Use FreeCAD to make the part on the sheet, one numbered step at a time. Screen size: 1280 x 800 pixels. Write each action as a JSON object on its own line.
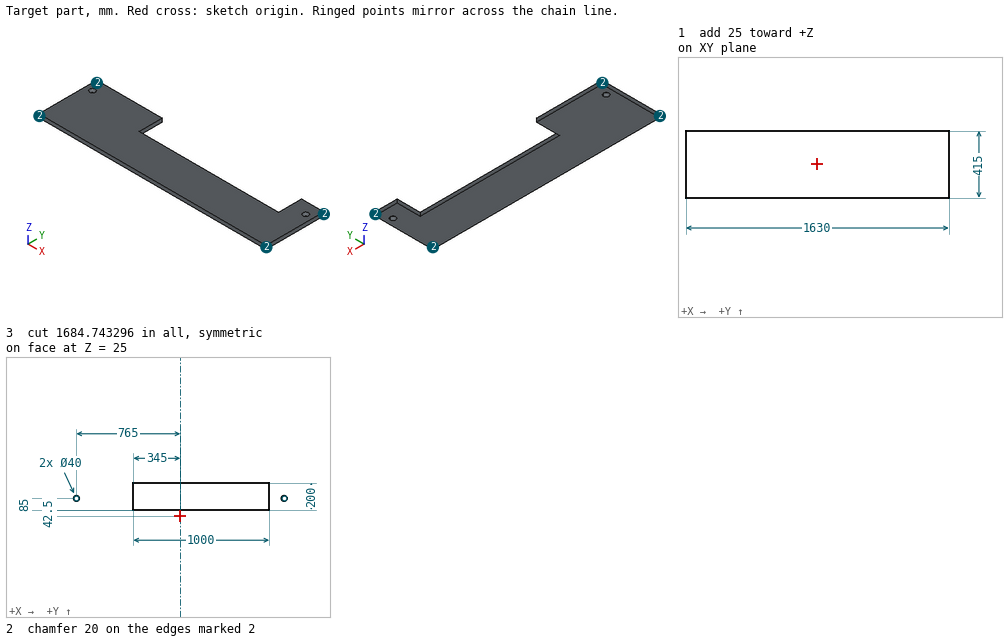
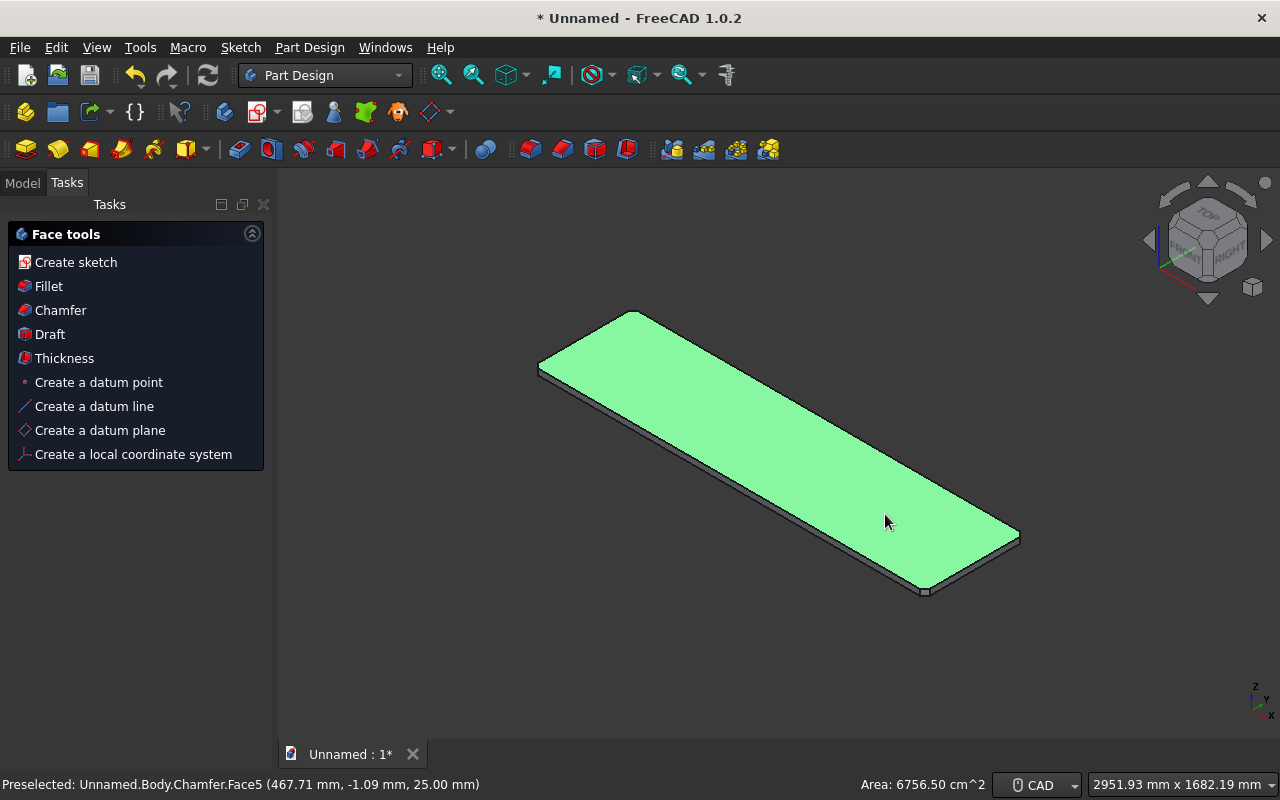
{"action": "left_click", "coordinate": [258, 112]}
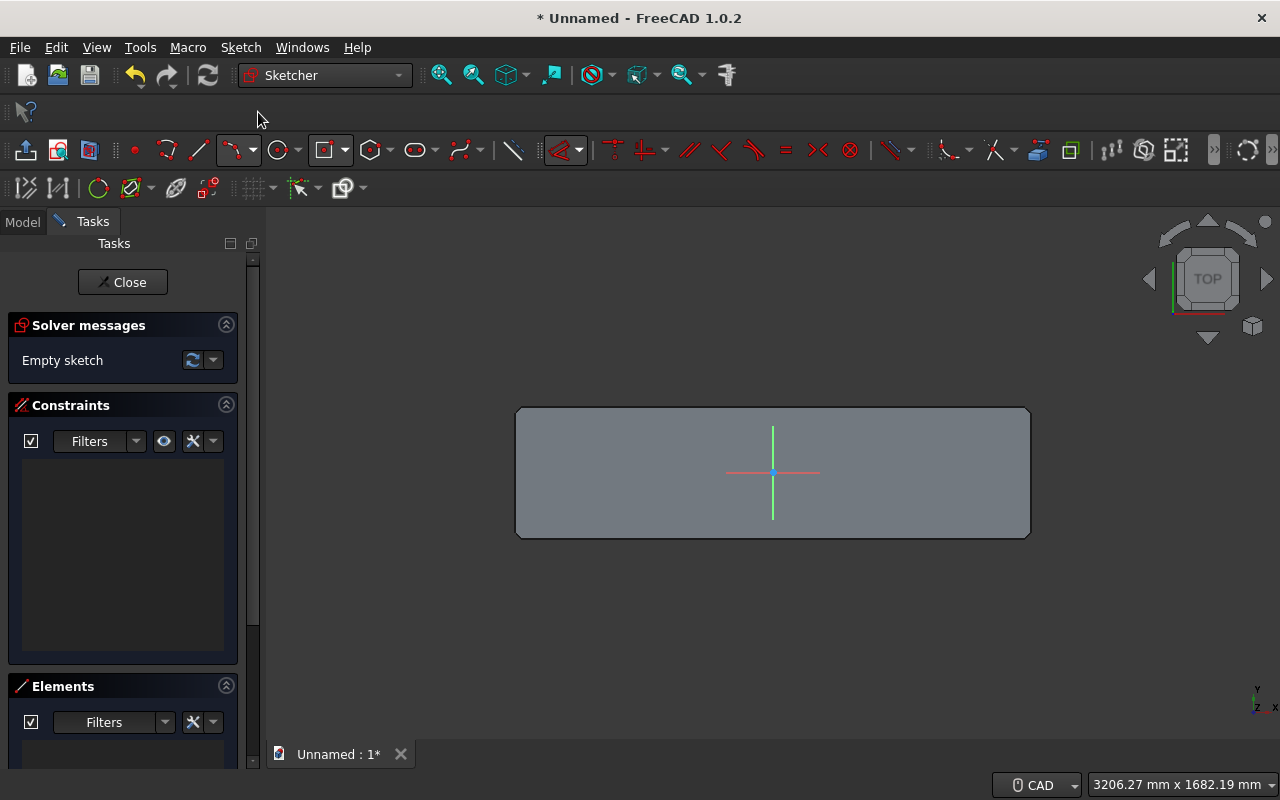
{"action": "key", "text": "g r"}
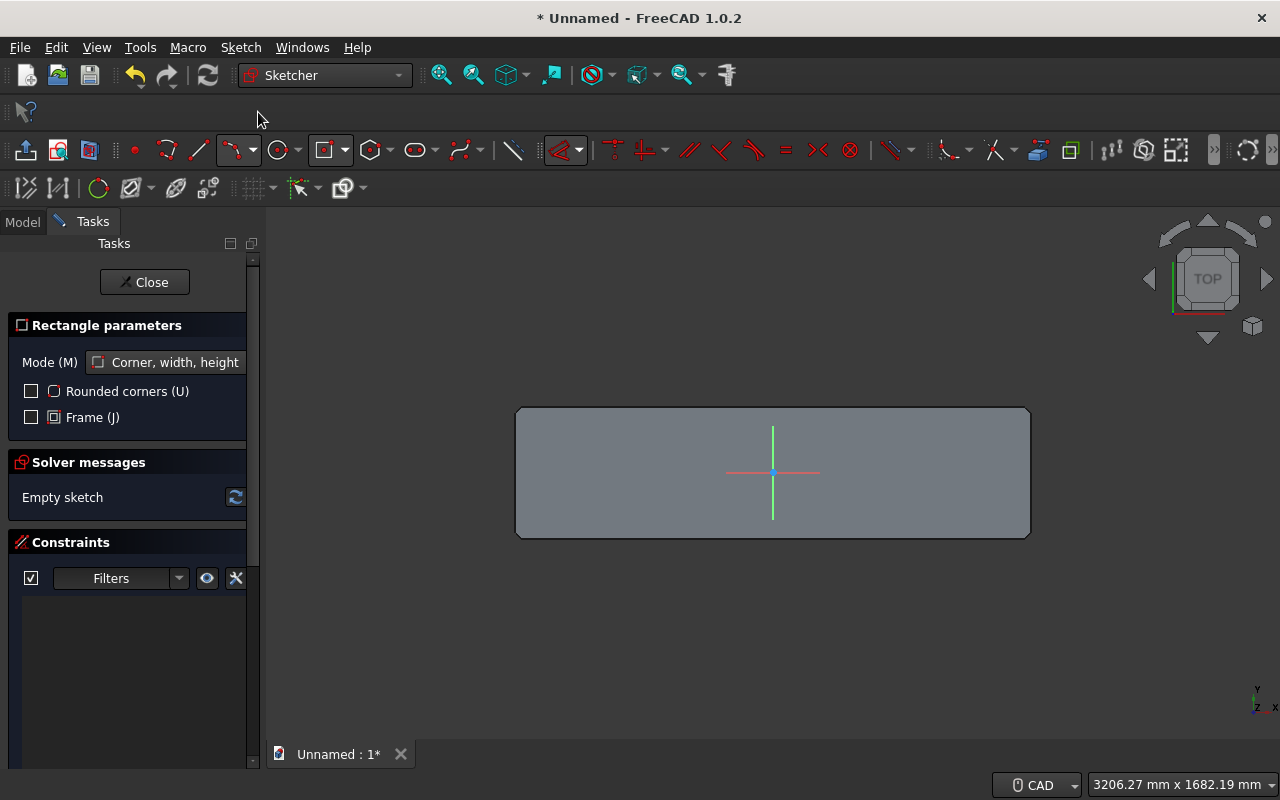
{"action": "left_click", "coordinate": [664, 396]}
{"action": "mouse_move", "coordinate": [980, 460]}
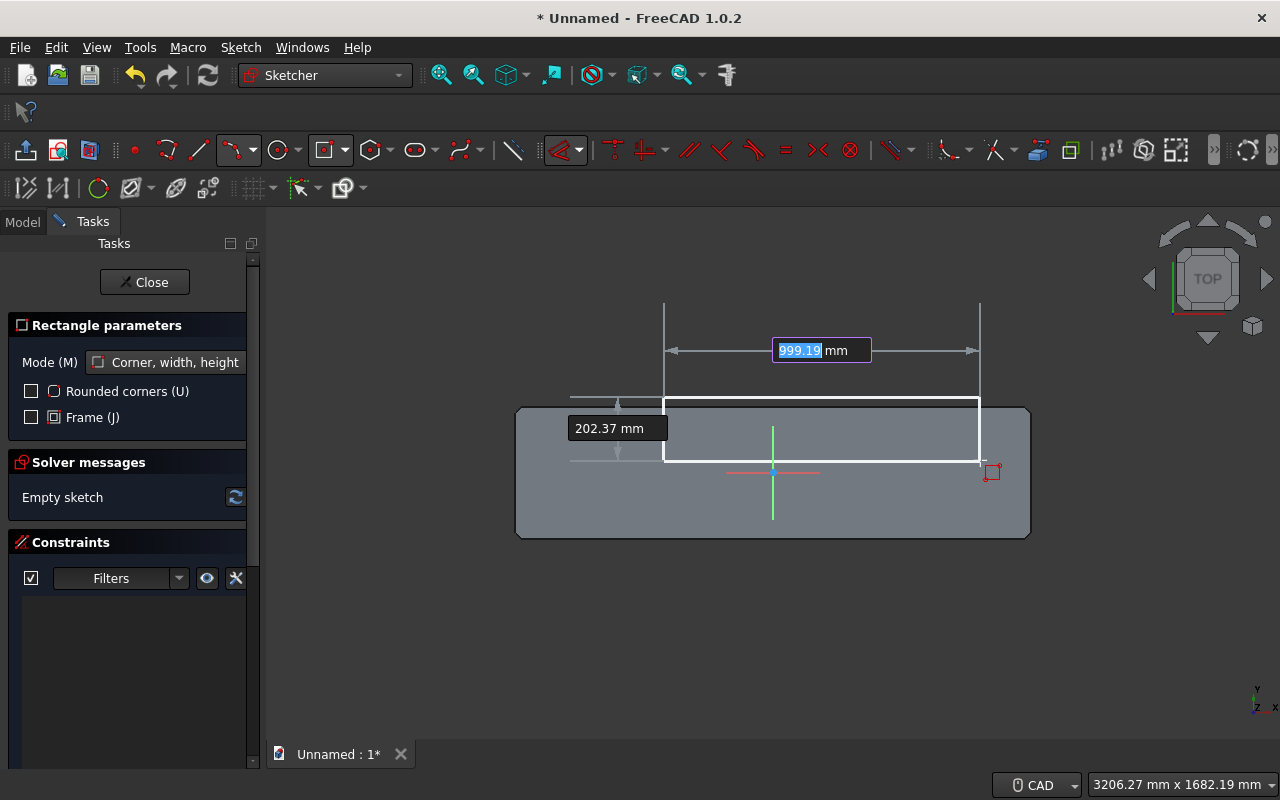
{"action": "type", "text": "1000"}
{"action": "key", "text": "Tab"}
{"action": "type", "text": "200"}
{"action": "key", "text": "Return"}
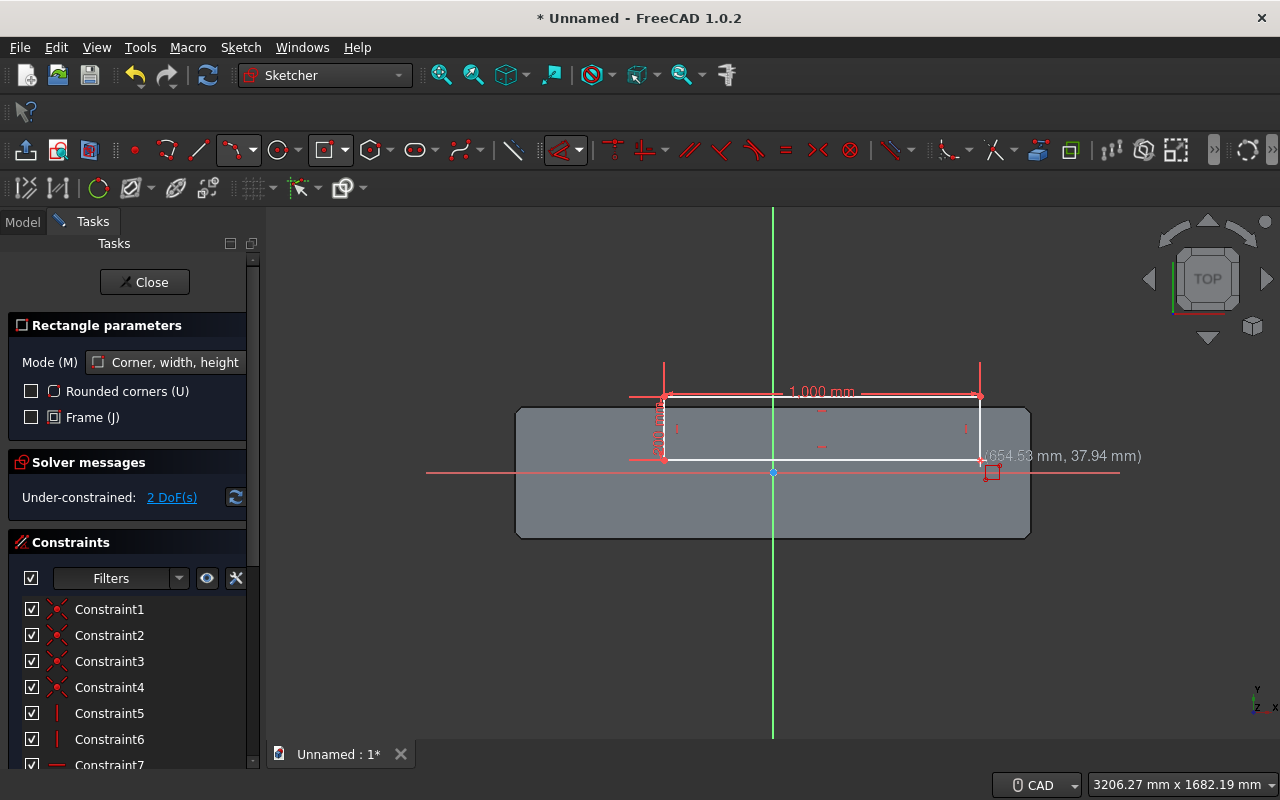
{"action": "left_click", "coordinate": [278, 150]}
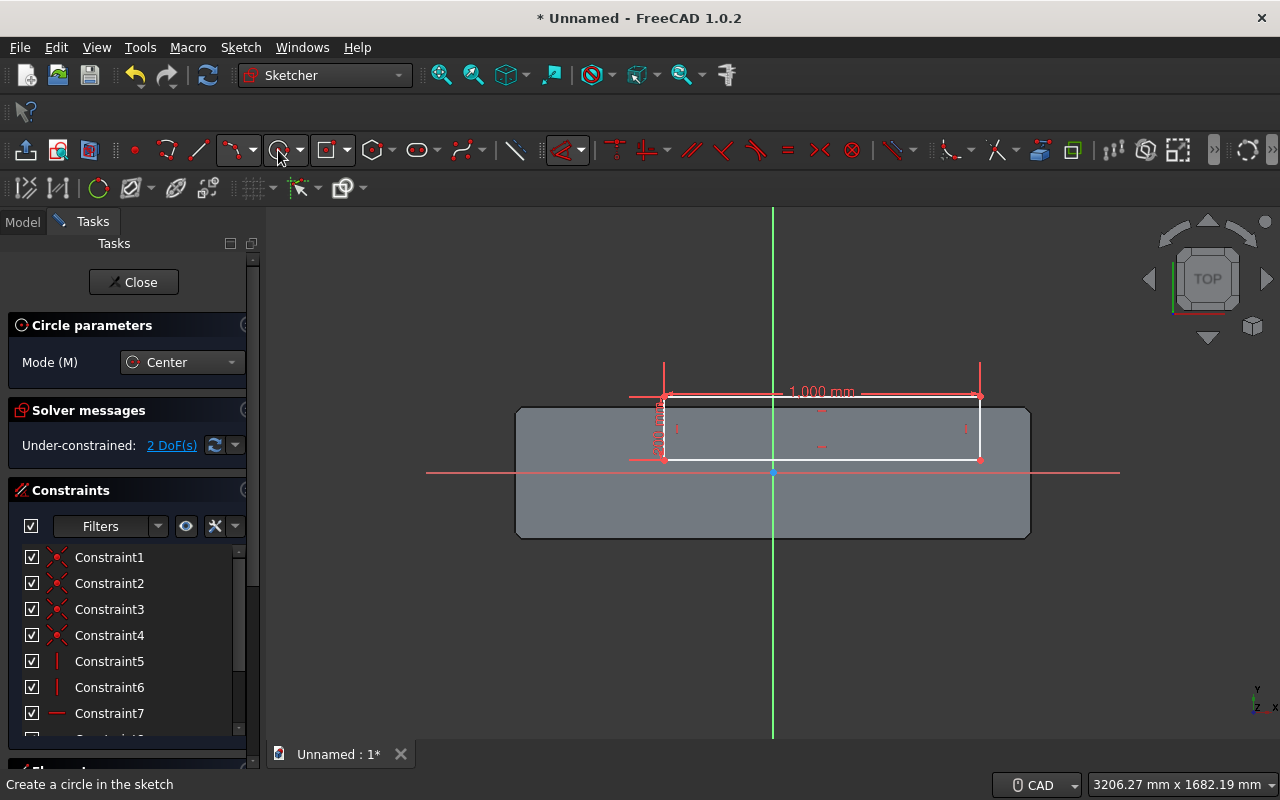
{"action": "scroll", "coordinate": [531, 433], "scroll_direction": "up", "scroll_amount": 7}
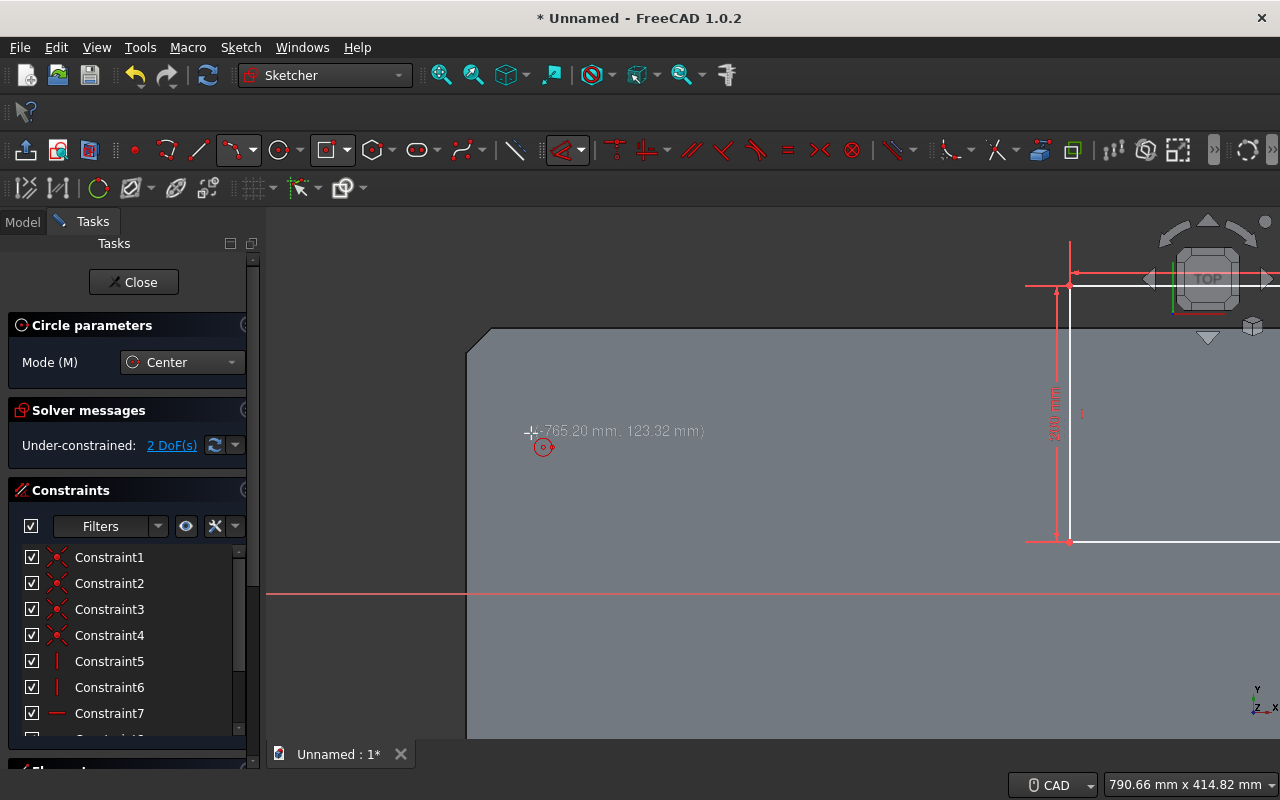
{"action": "scroll", "coordinate": [357, 488], "scroll_direction": "down", "scroll_amount": 6}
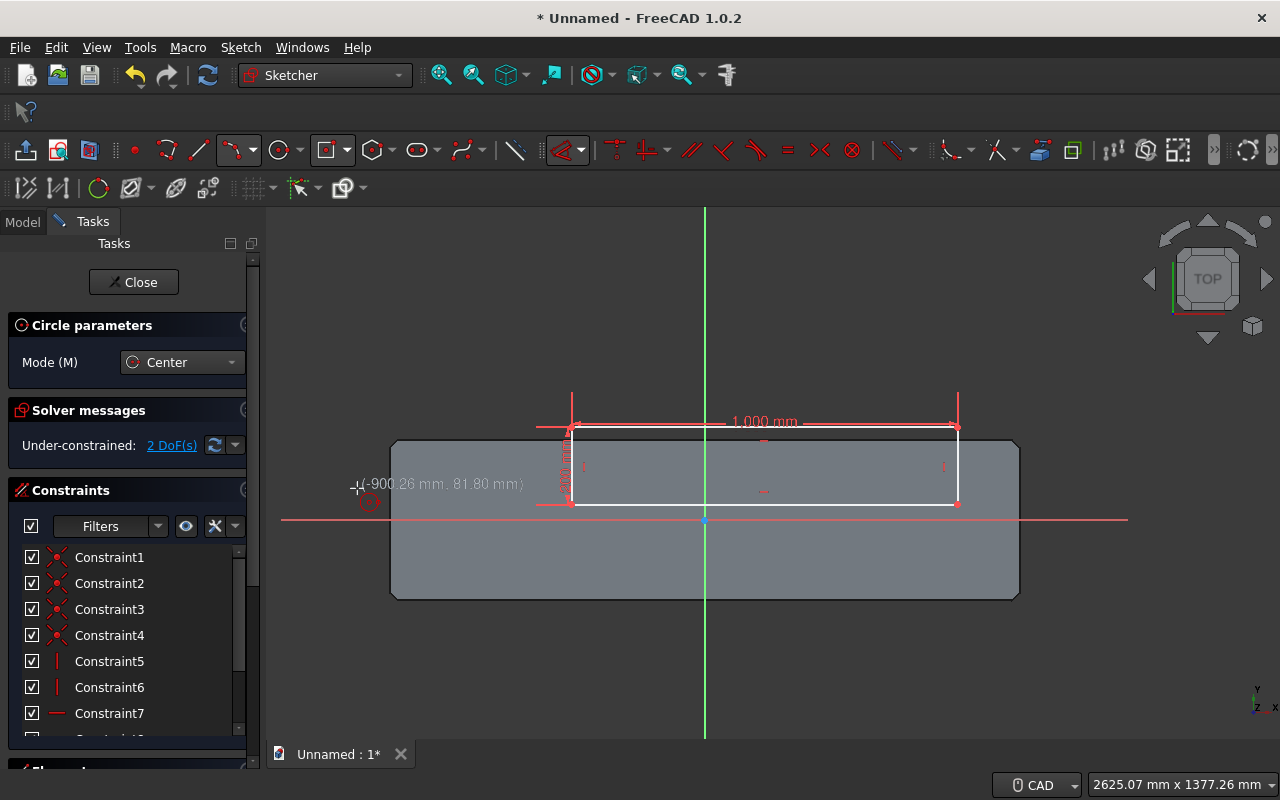
{"action": "left_click", "coordinate": [409, 471]}
{"action": "mouse_move", "coordinate": [415, 466]}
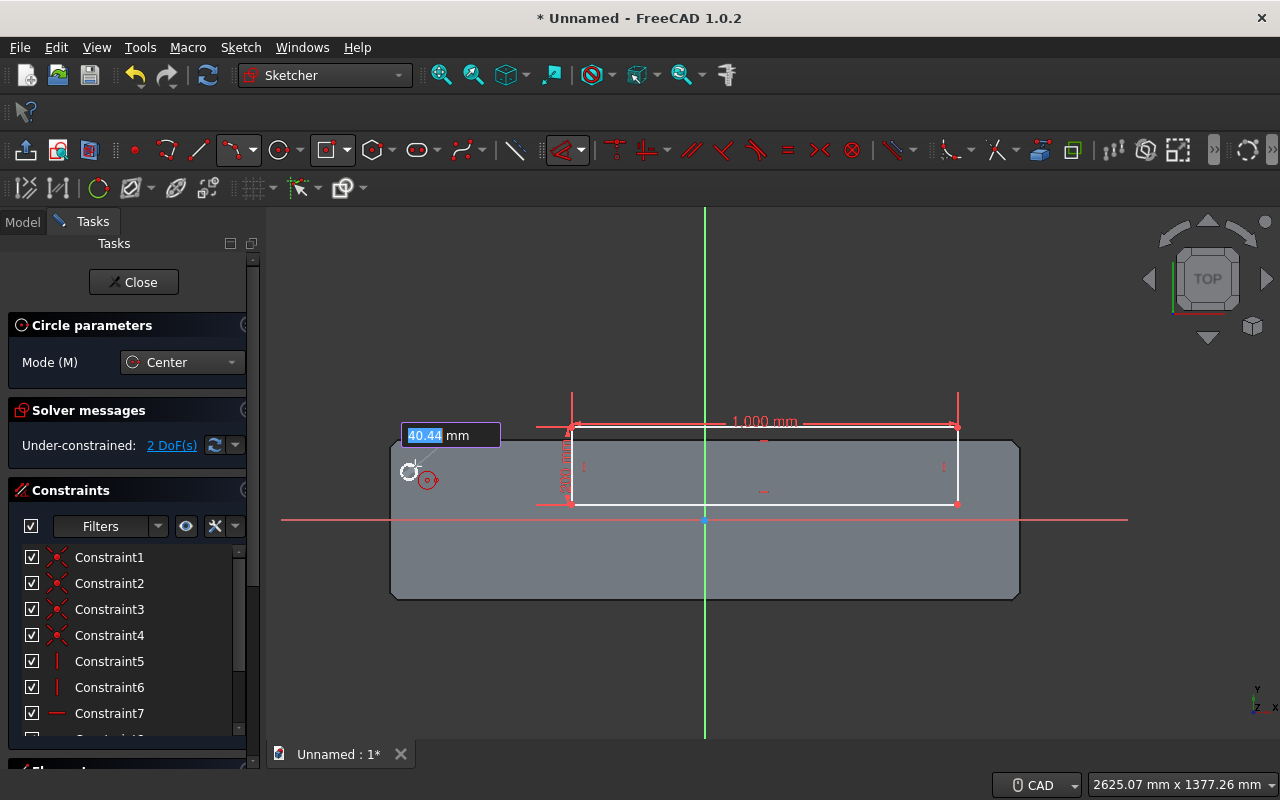
{"action": "type", "text": "40"}
{"action": "key", "text": "Return"}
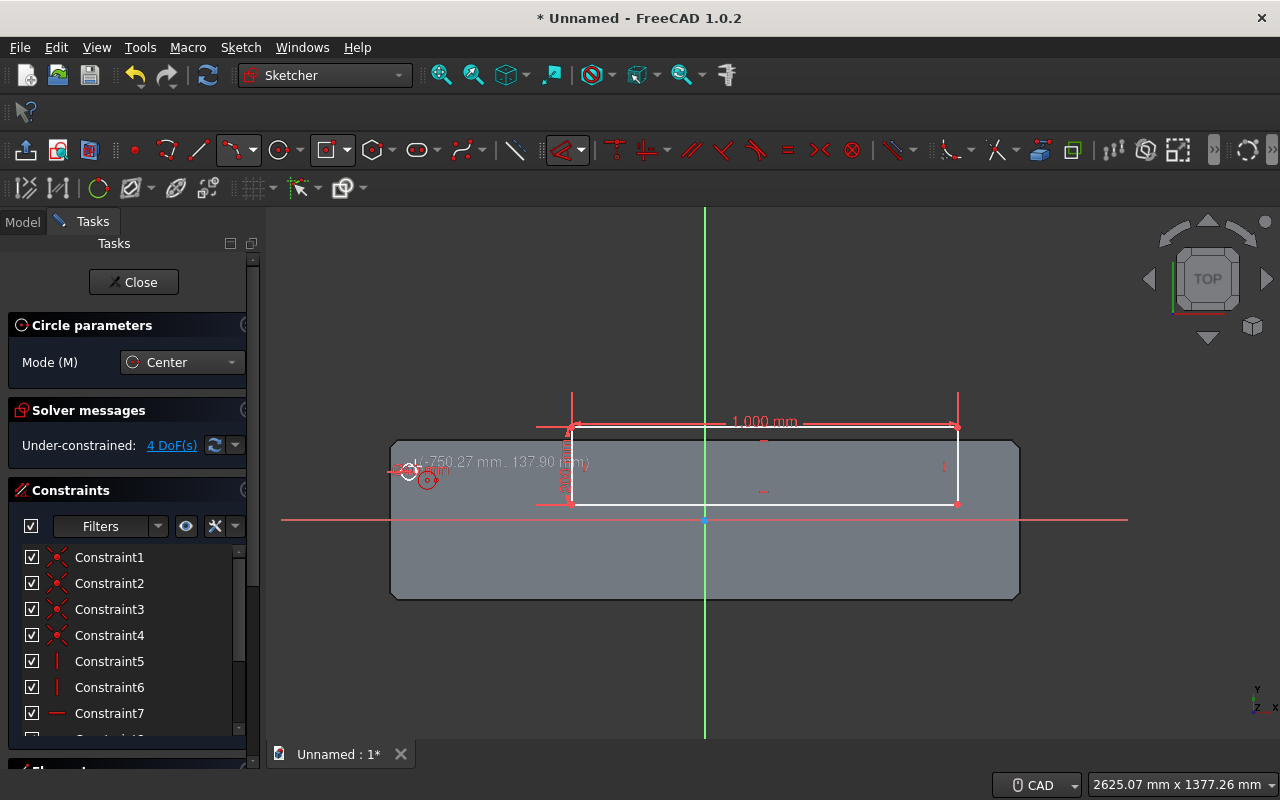
{"action": "scroll", "coordinate": [1000, 471], "scroll_direction": "up", "scroll_amount": 6}